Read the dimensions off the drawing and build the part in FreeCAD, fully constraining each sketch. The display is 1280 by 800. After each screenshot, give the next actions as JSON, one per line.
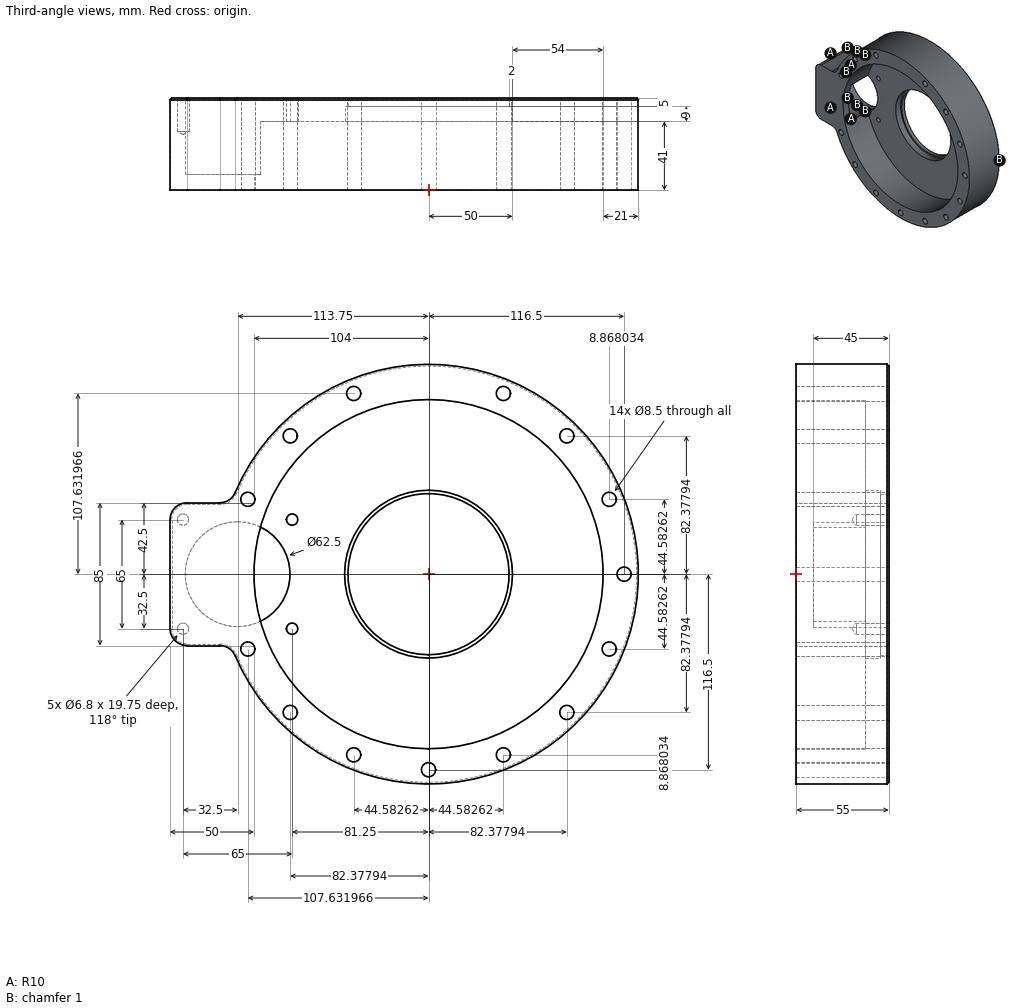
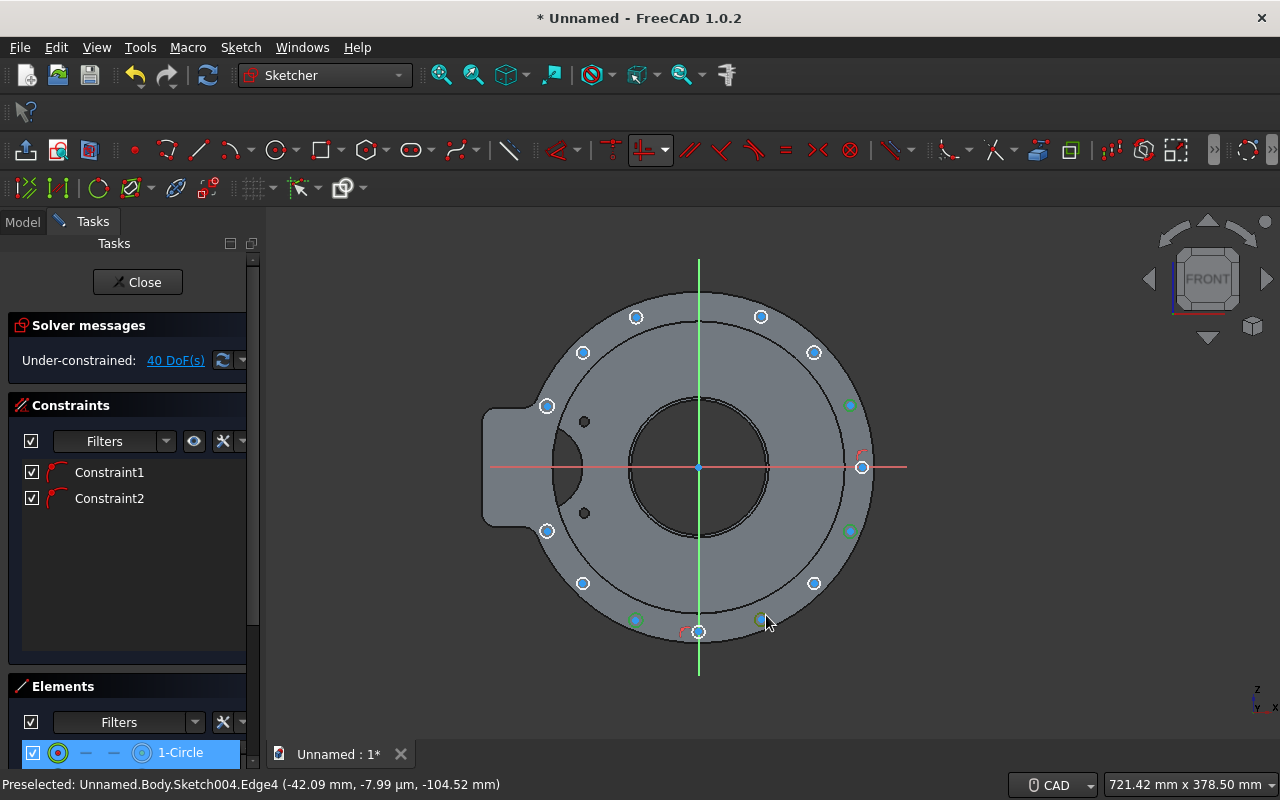
{"action": "scroll", "coordinate": [552, 526], "scroll_direction": "up", "scroll_amount": 4}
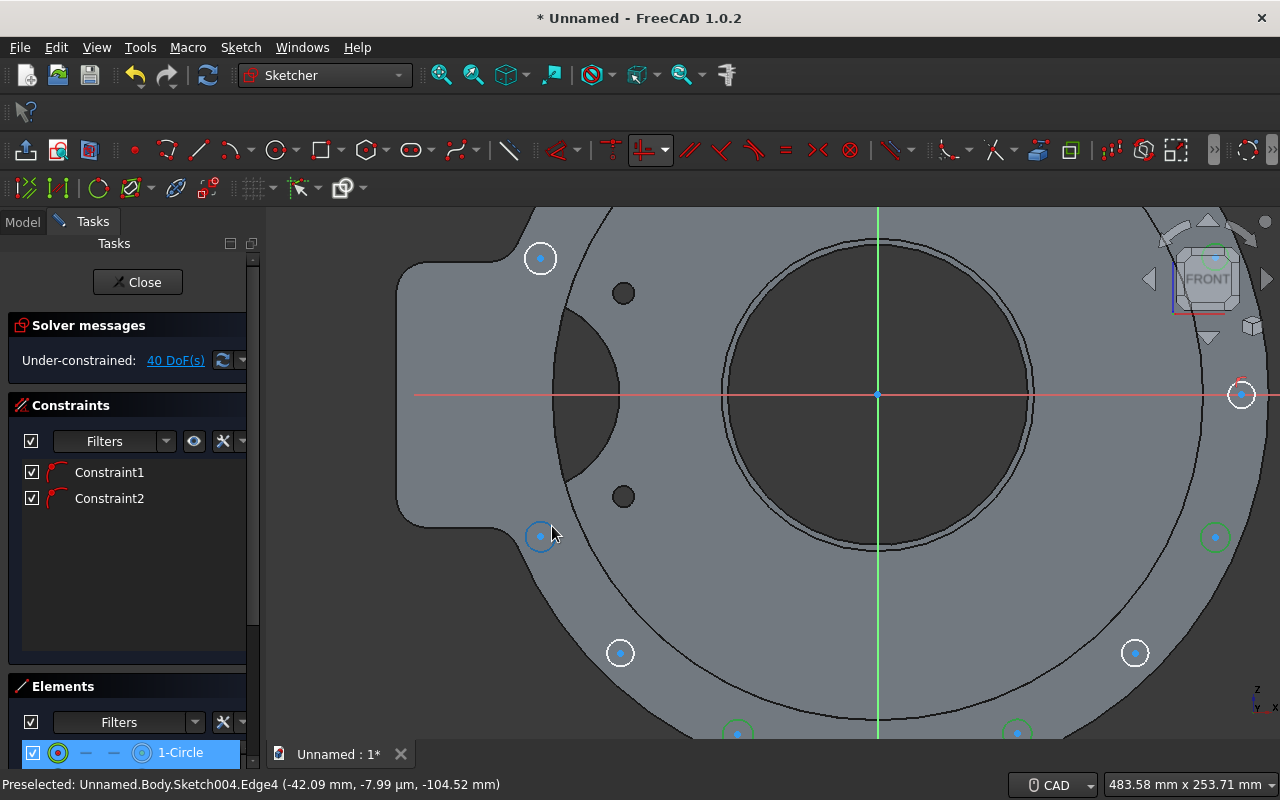
{"action": "left_click", "coordinate": [551, 526]}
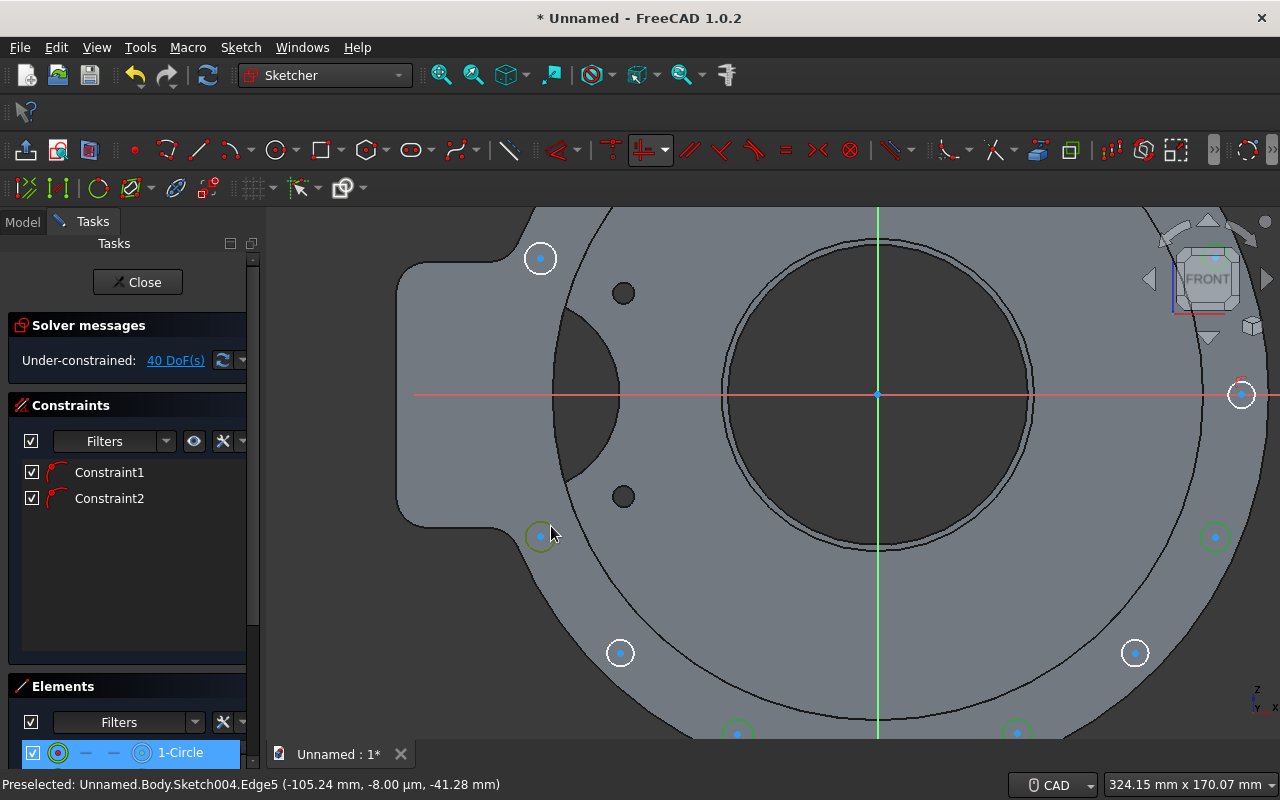
{"action": "left_click", "coordinate": [552, 247]}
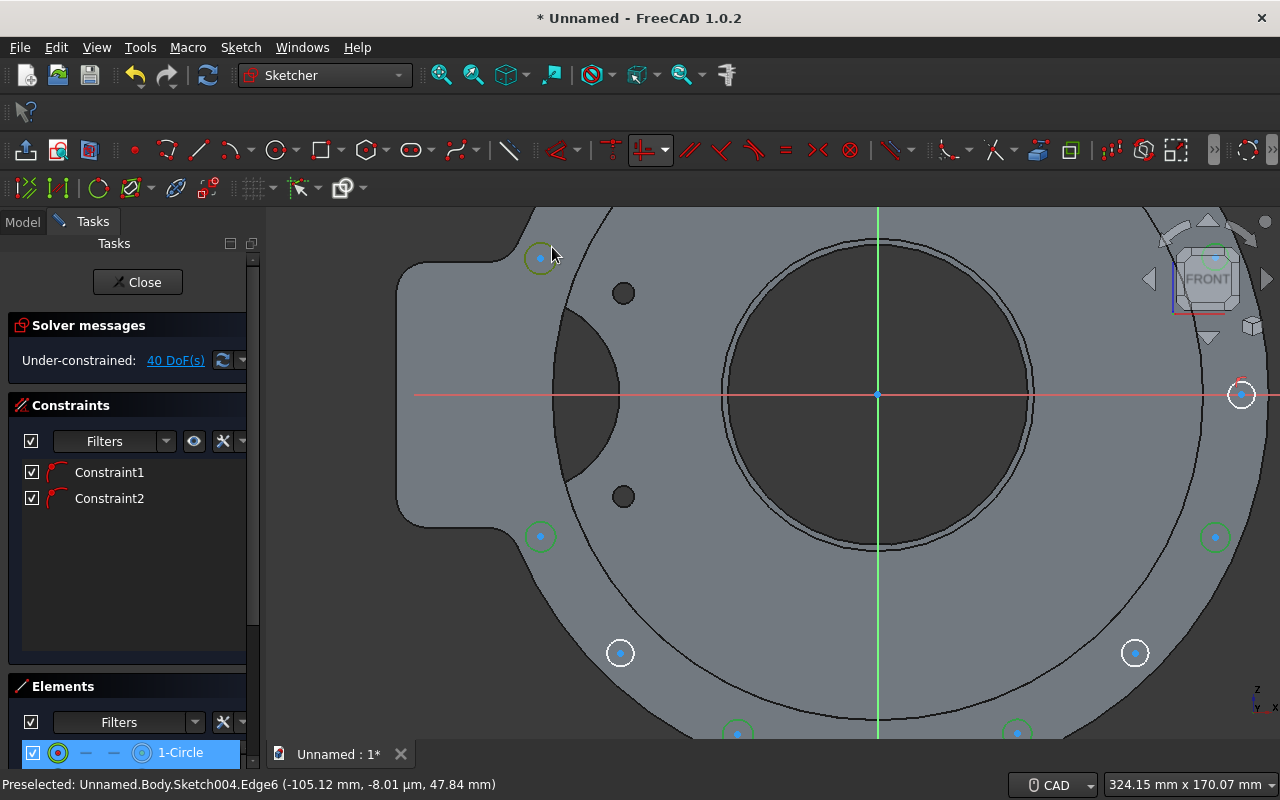
{"action": "scroll", "coordinate": [552, 525], "scroll_direction": "down", "scroll_amount": 4}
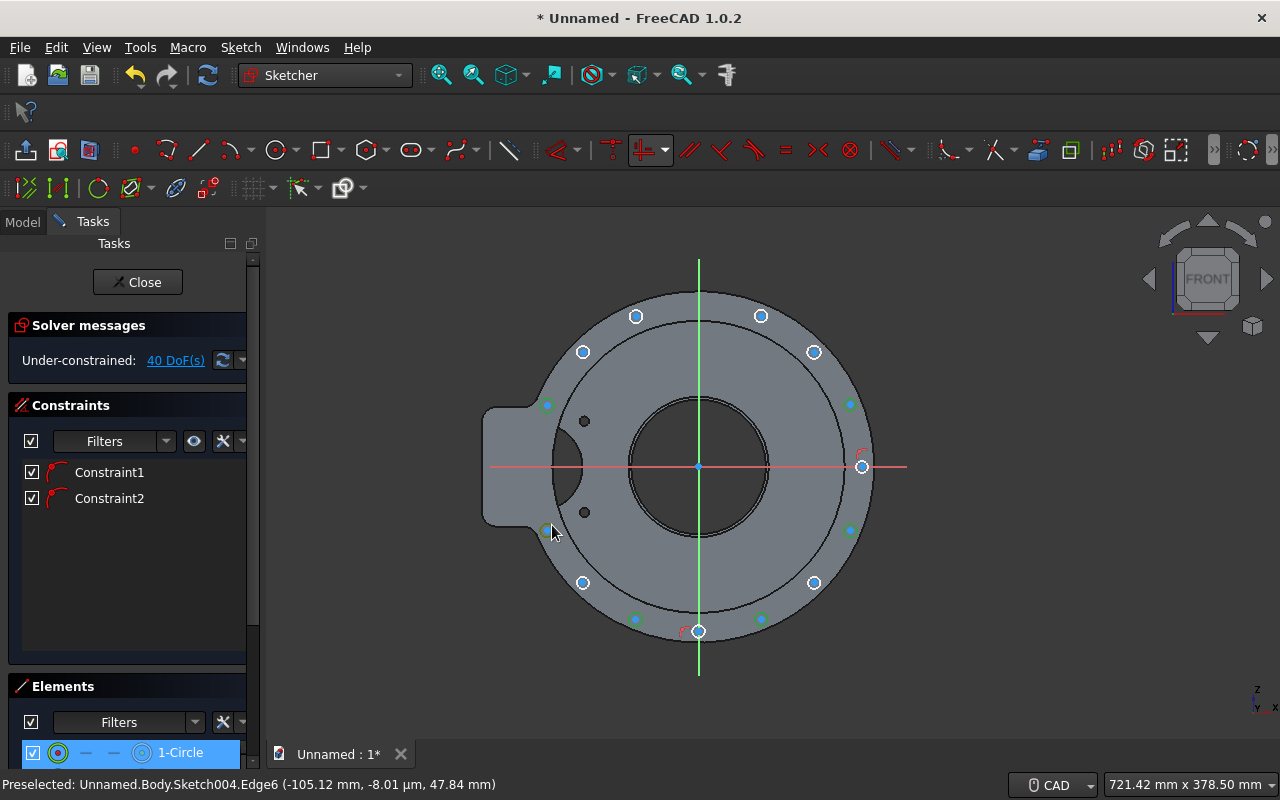
{"action": "scroll", "coordinate": [641, 312], "scroll_direction": "up", "scroll_amount": 4}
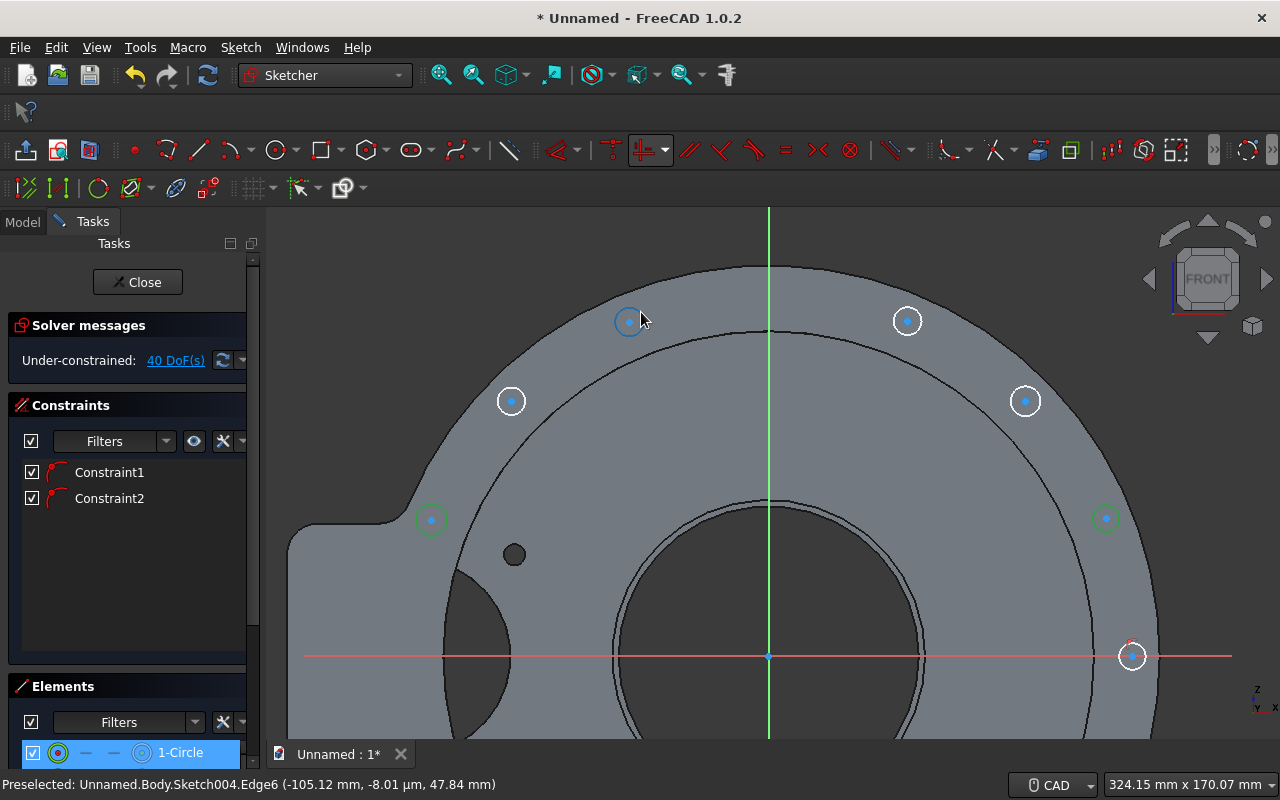
{"action": "left_click", "coordinate": [640, 312]}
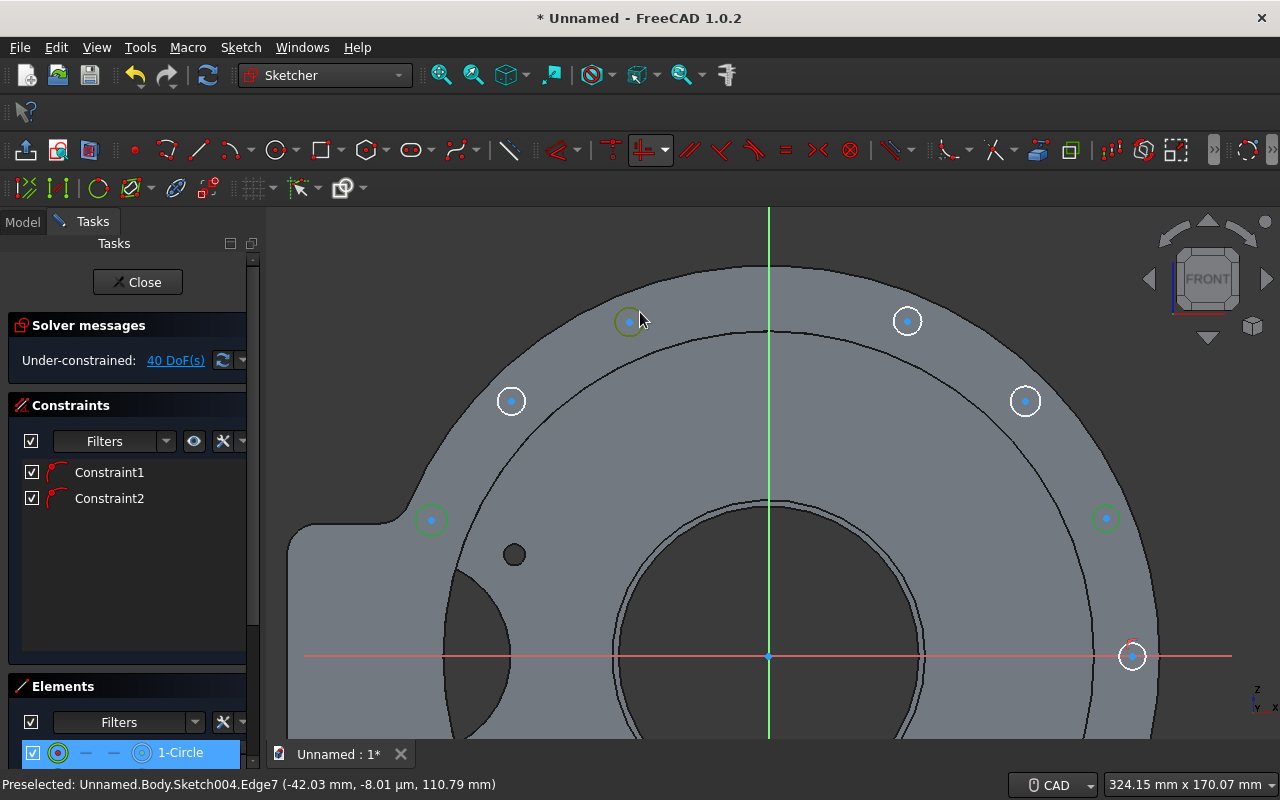
{"action": "left_click", "coordinate": [917, 311]}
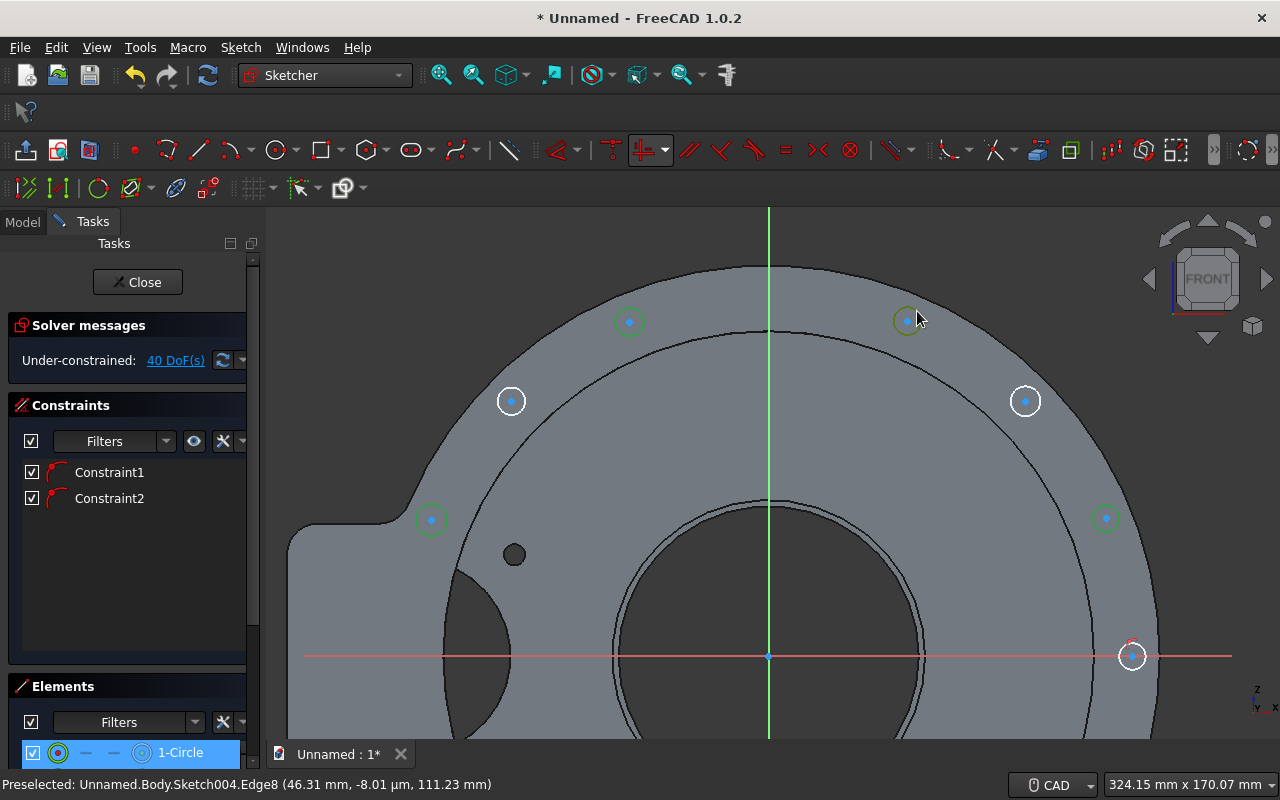
{"action": "scroll", "coordinate": [641, 312], "scroll_direction": "down", "scroll_amount": 4}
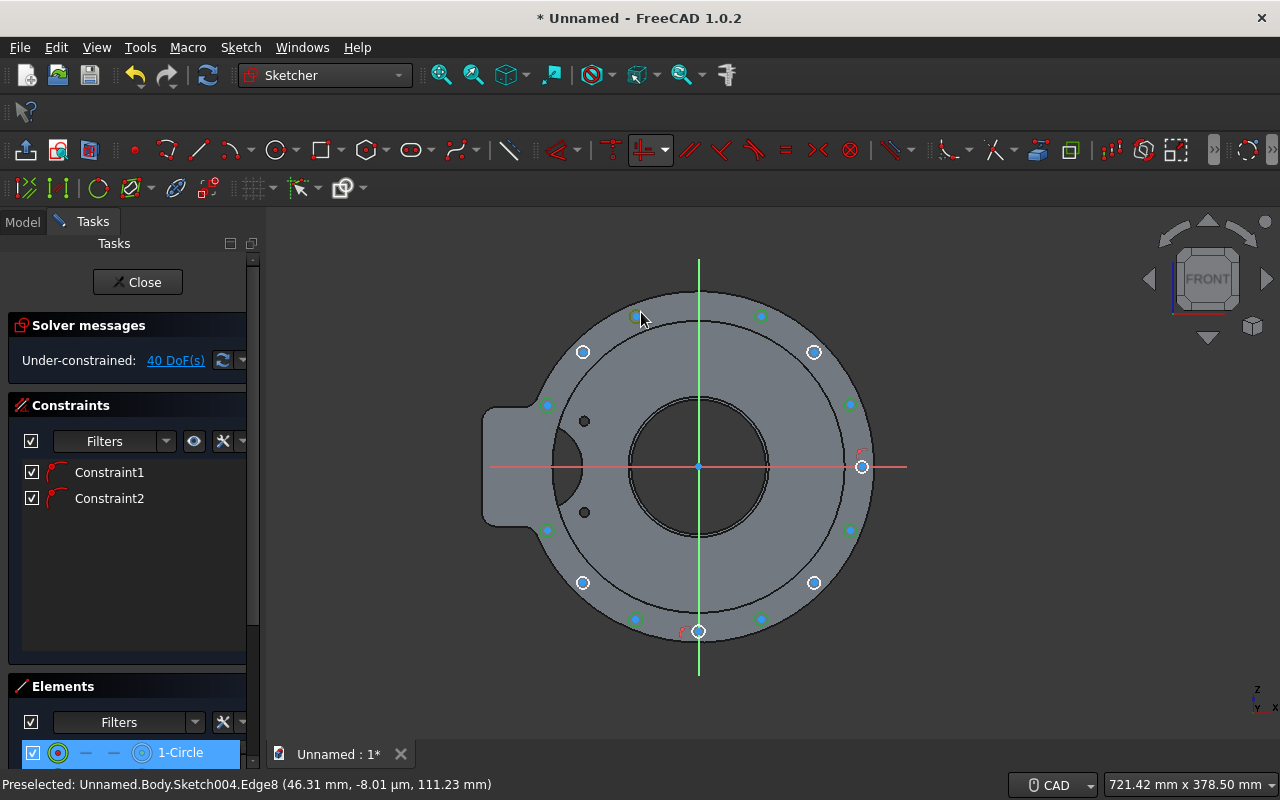
{"action": "scroll", "coordinate": [703, 627], "scroll_direction": "up", "scroll_amount": 6}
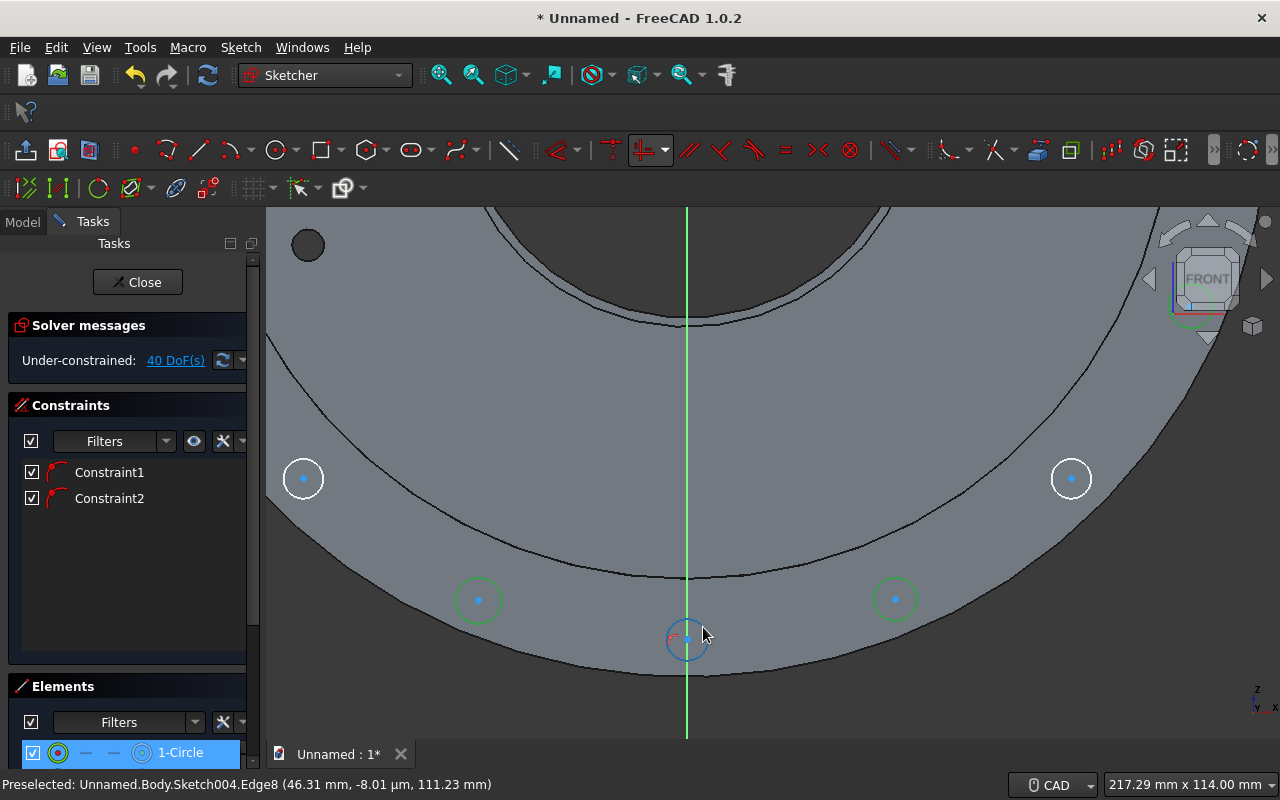
{"action": "left_click", "coordinate": [702, 625]}